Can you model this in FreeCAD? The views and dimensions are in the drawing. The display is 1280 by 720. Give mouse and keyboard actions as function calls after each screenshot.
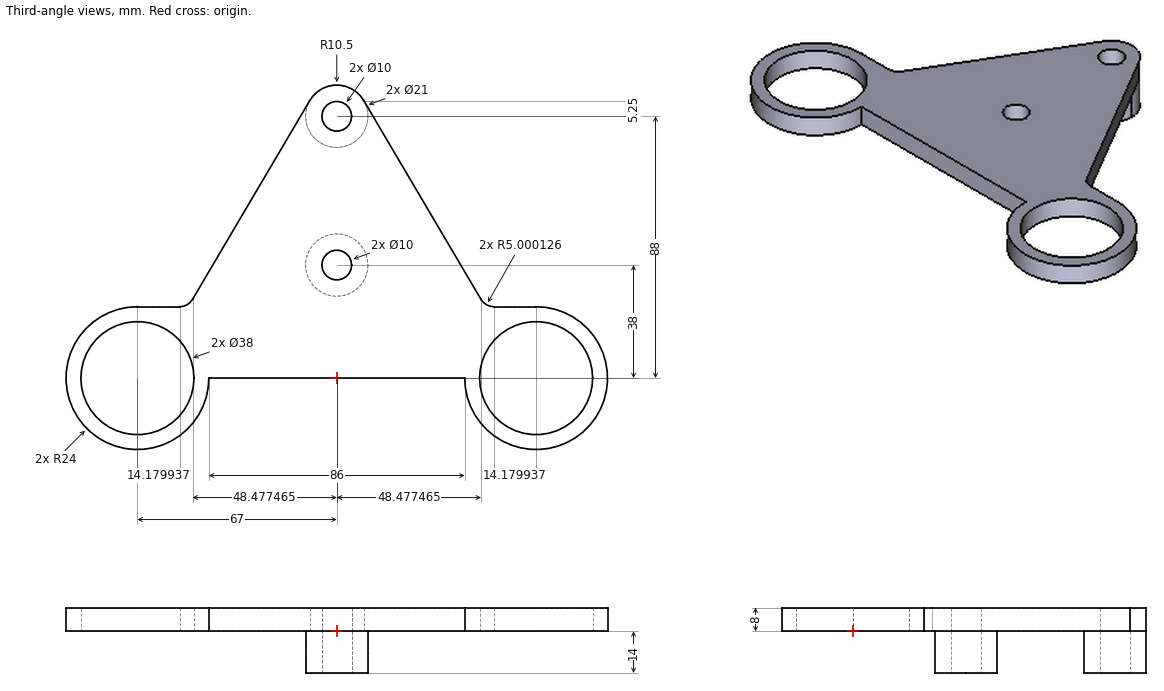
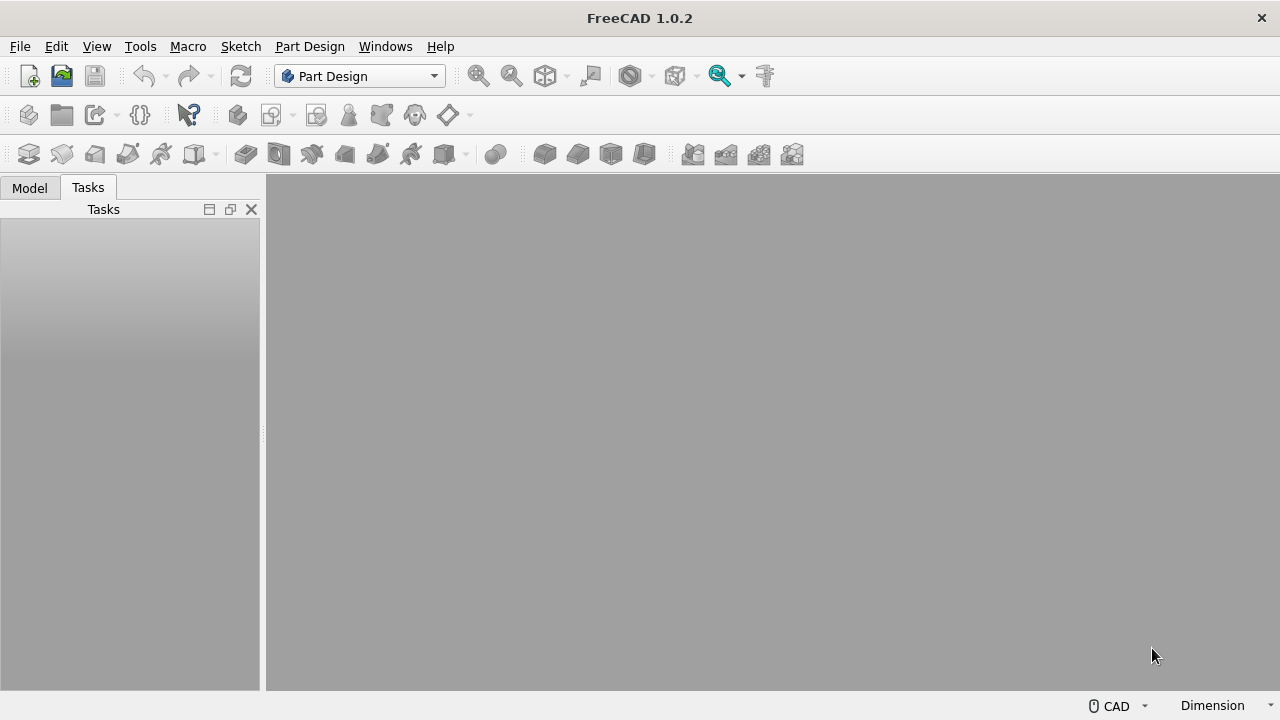
click(29, 76)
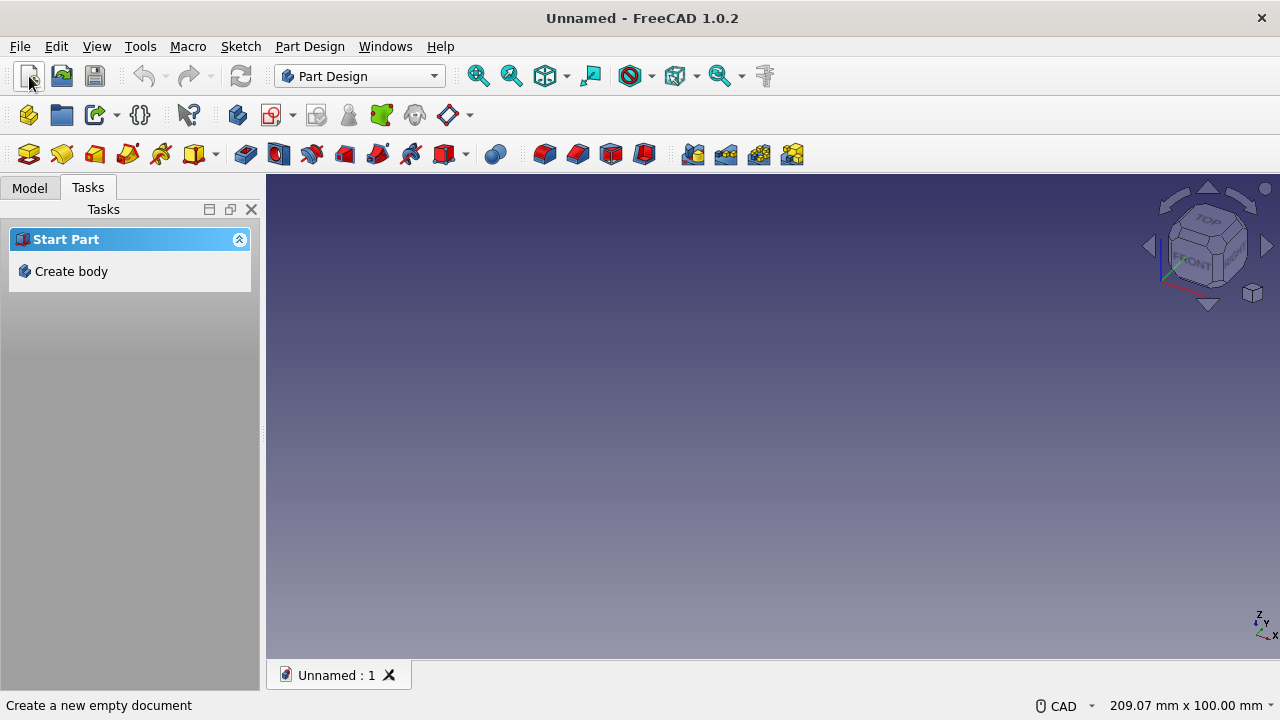
click(270, 116)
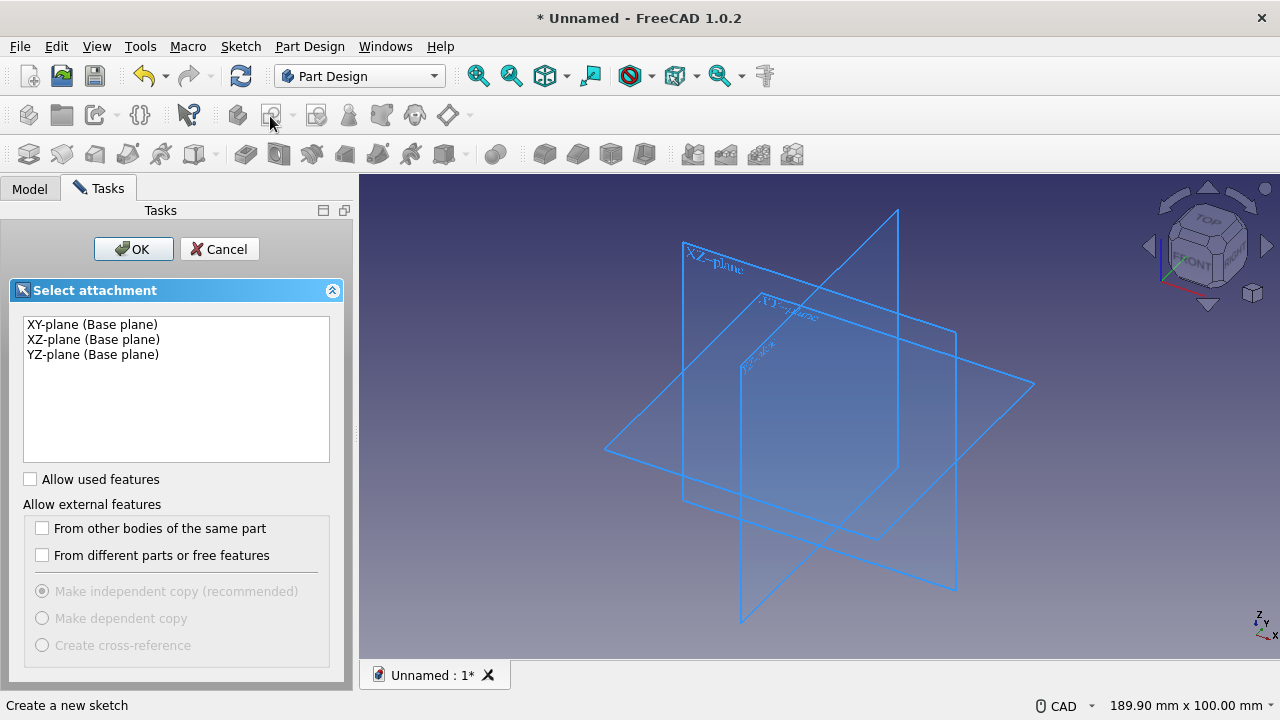
click(84, 324)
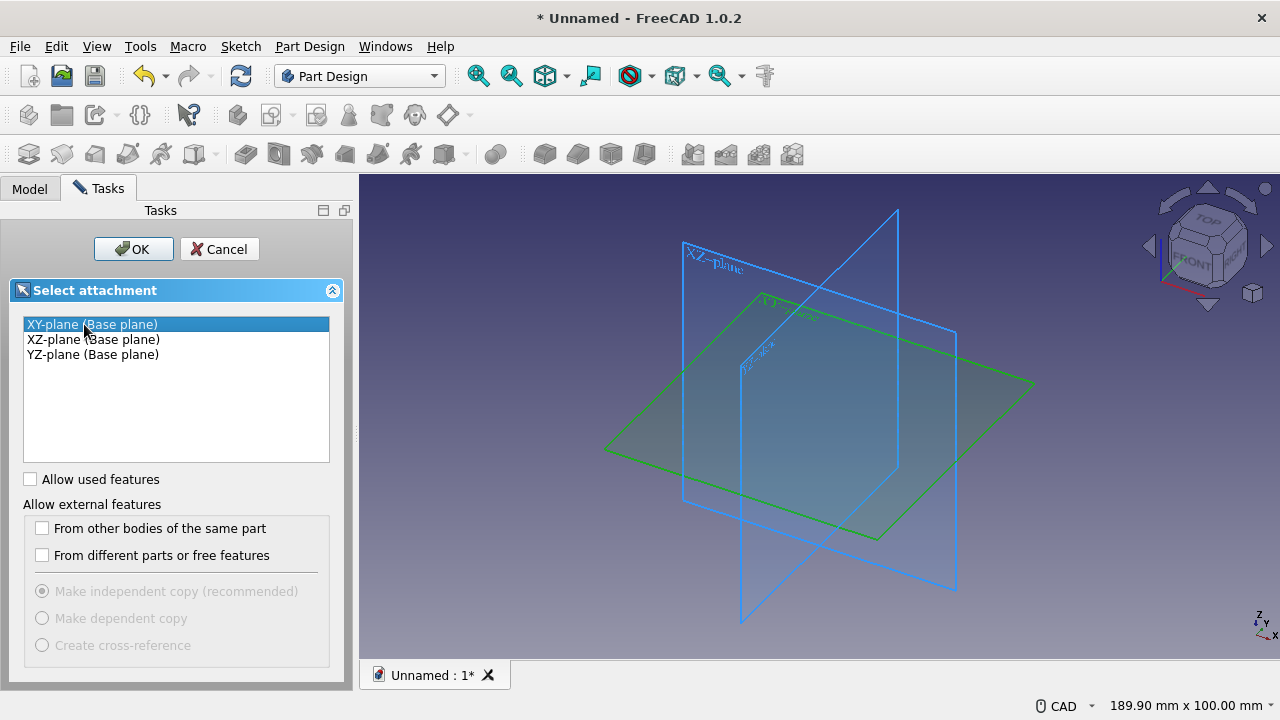
click(134, 249)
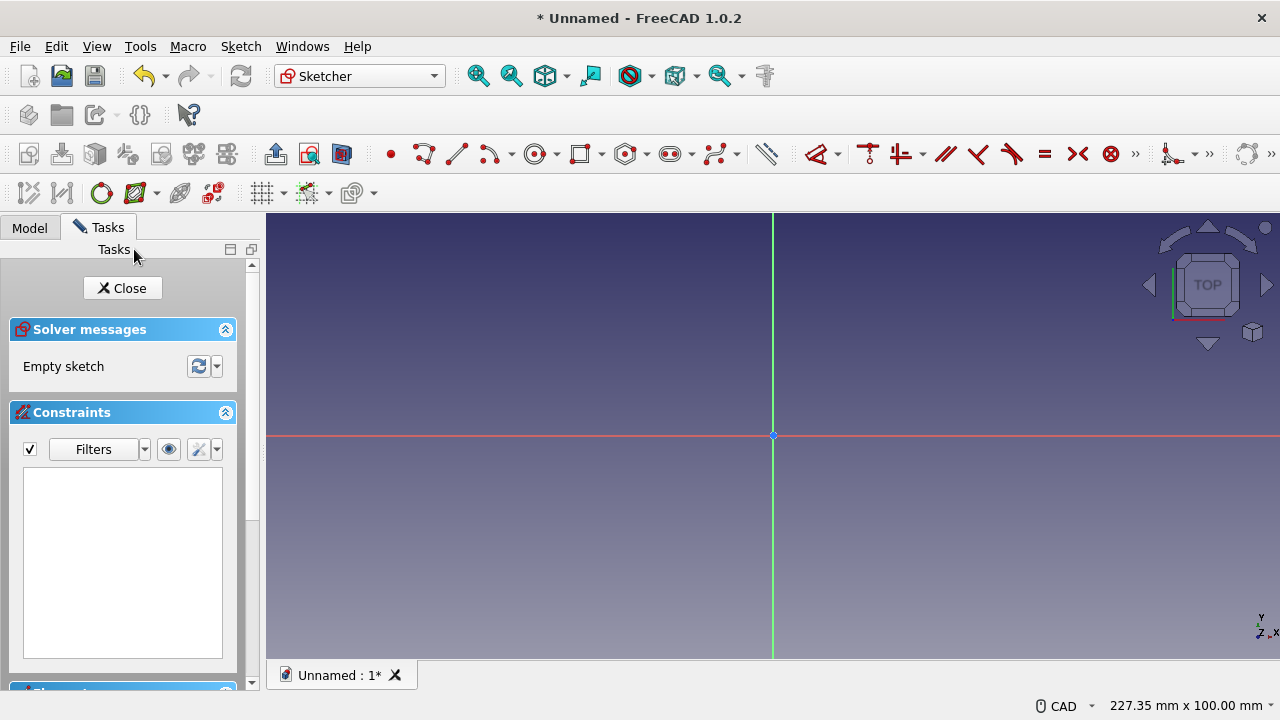
scroll(621, 631, down, 3)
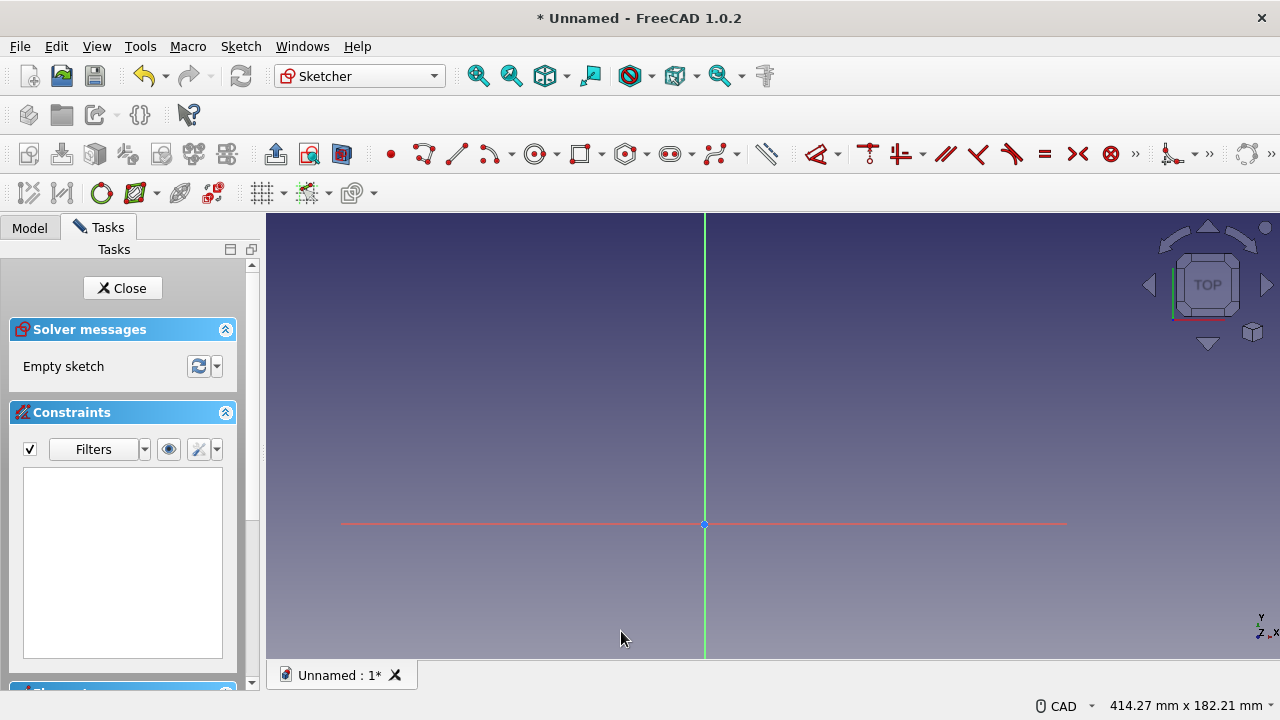
click(457, 154)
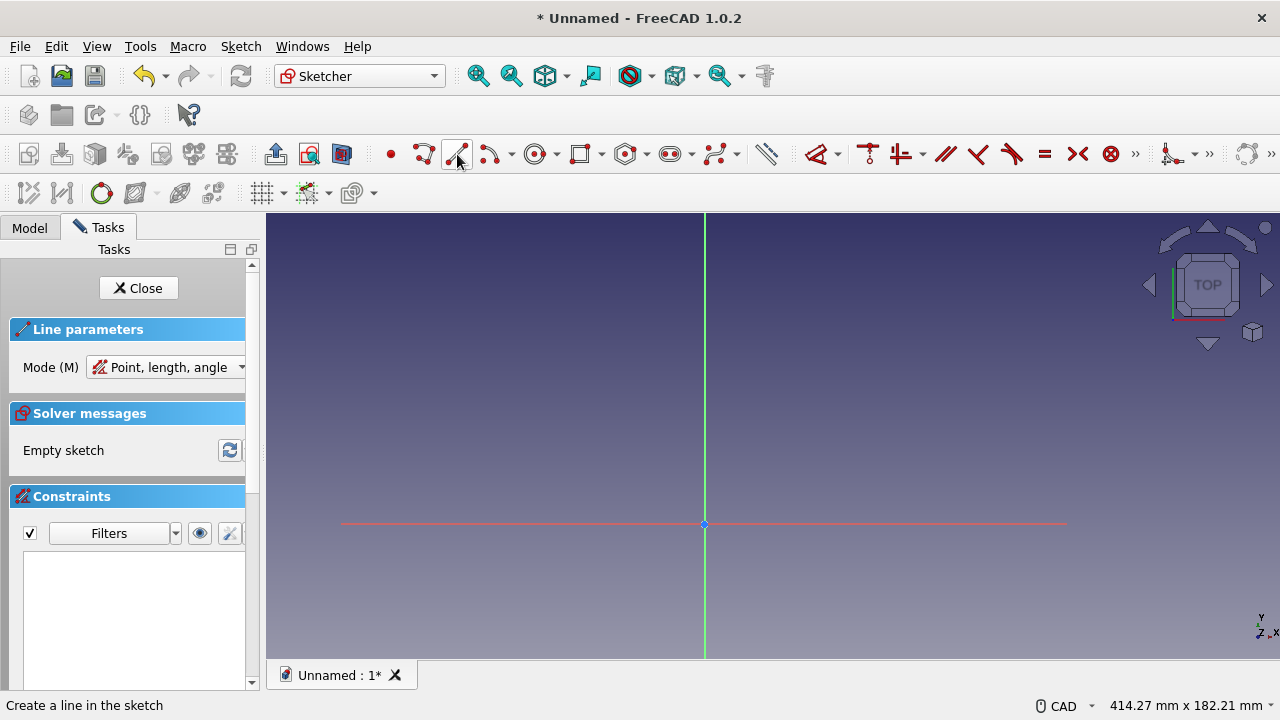
click(599, 524)
click(810, 515)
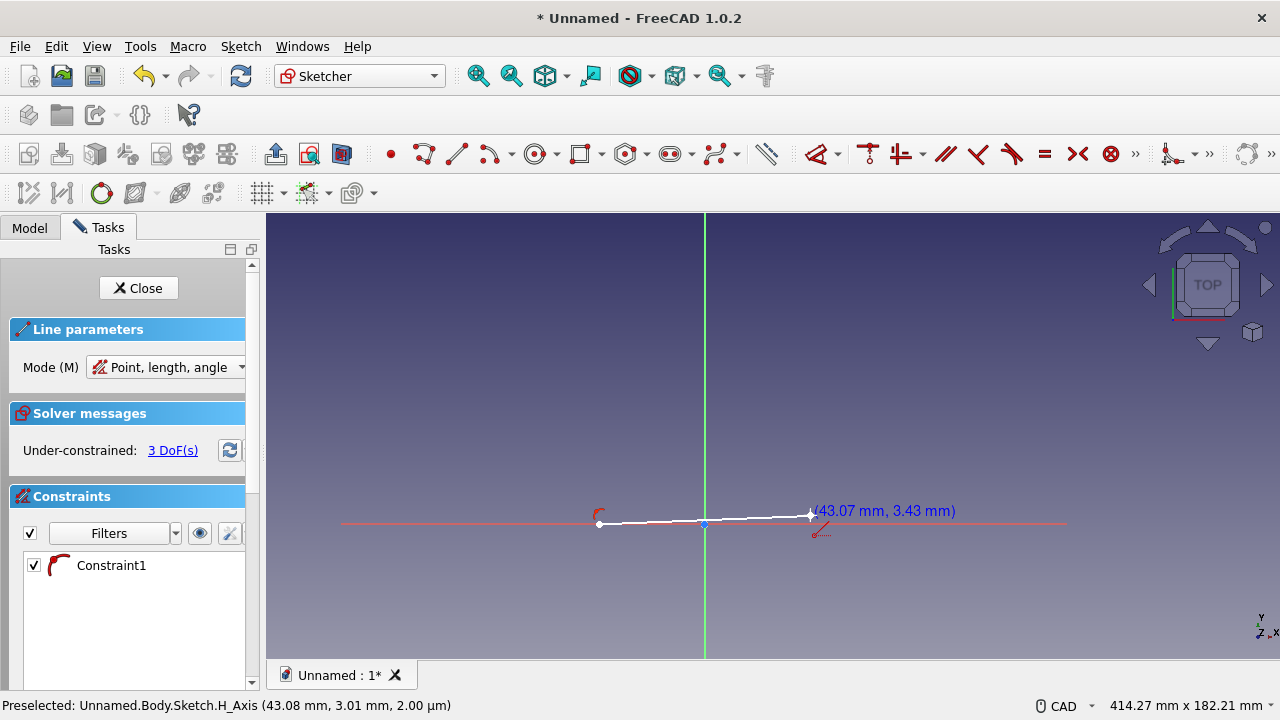
click(869, 466)
click(834, 466)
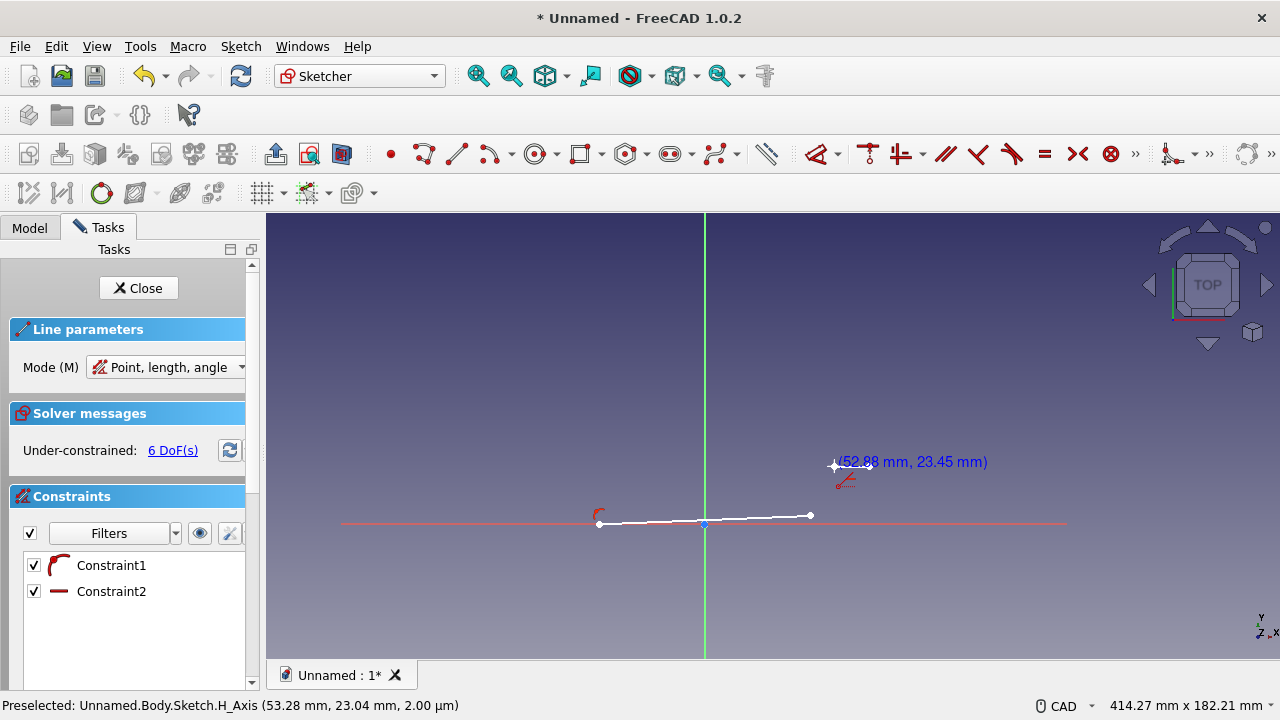
scroll(823, 460, up, 2)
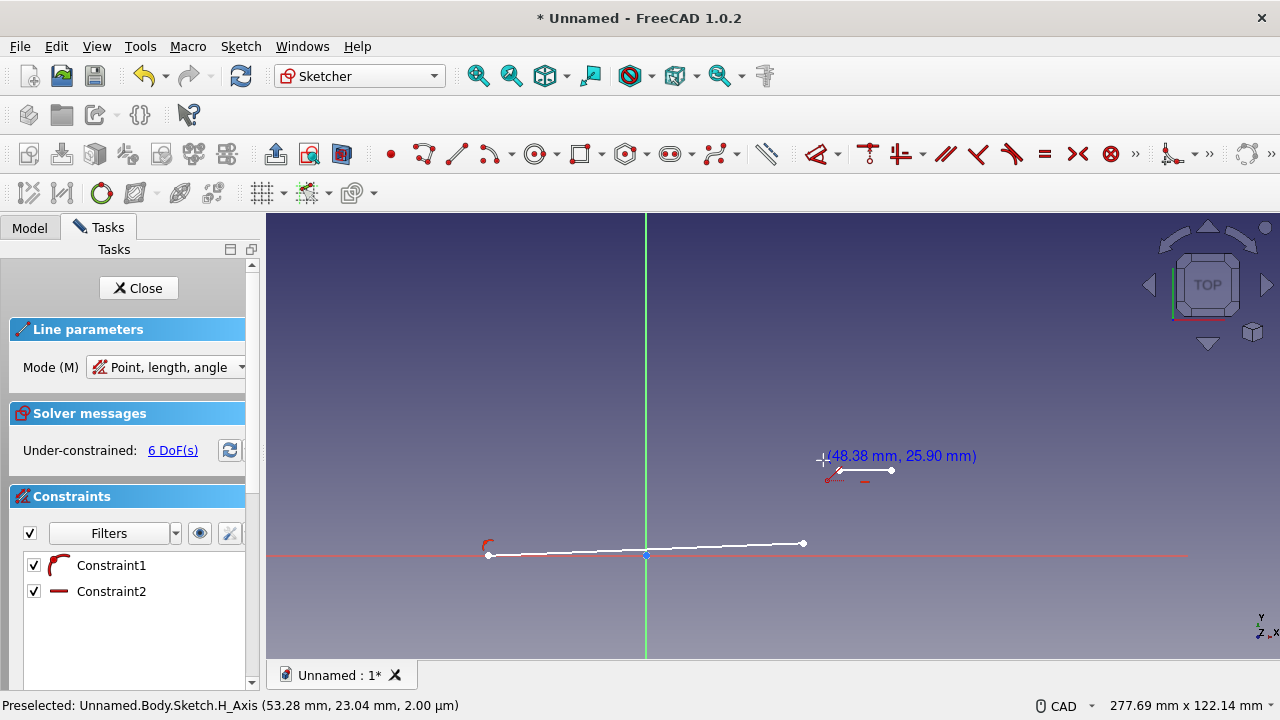
click(823, 459)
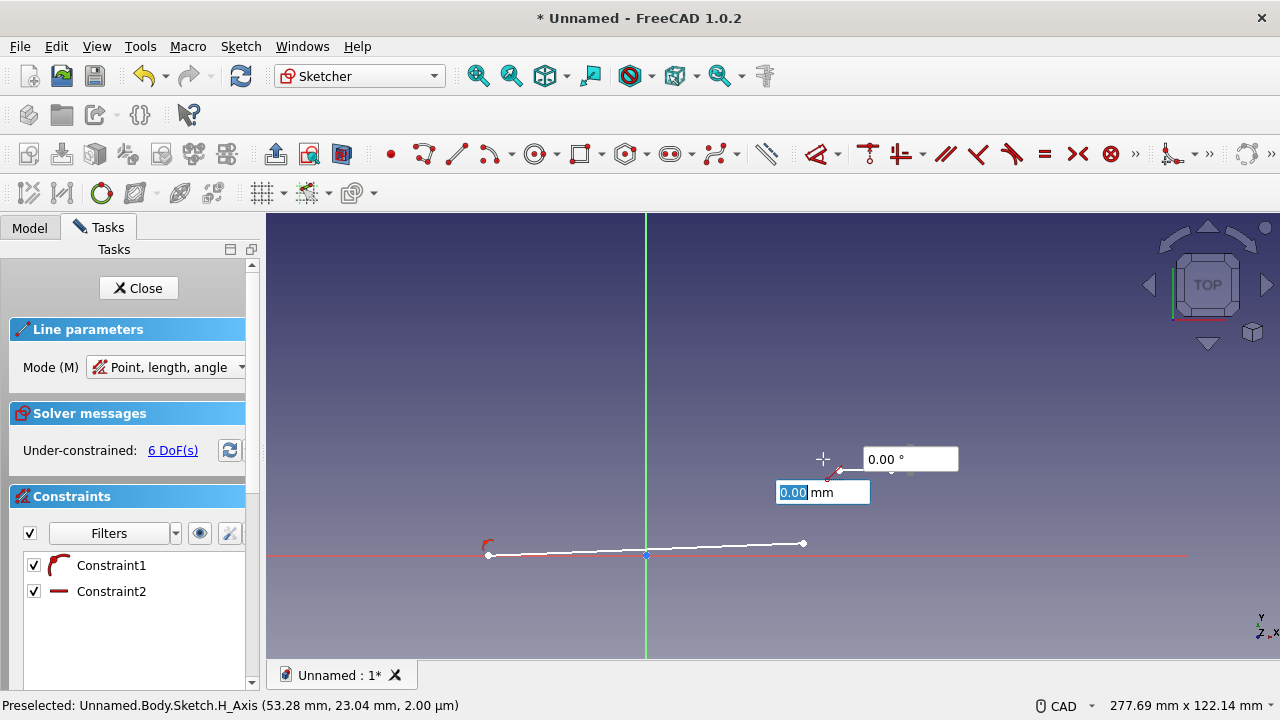
scroll(823, 488, down, 2)